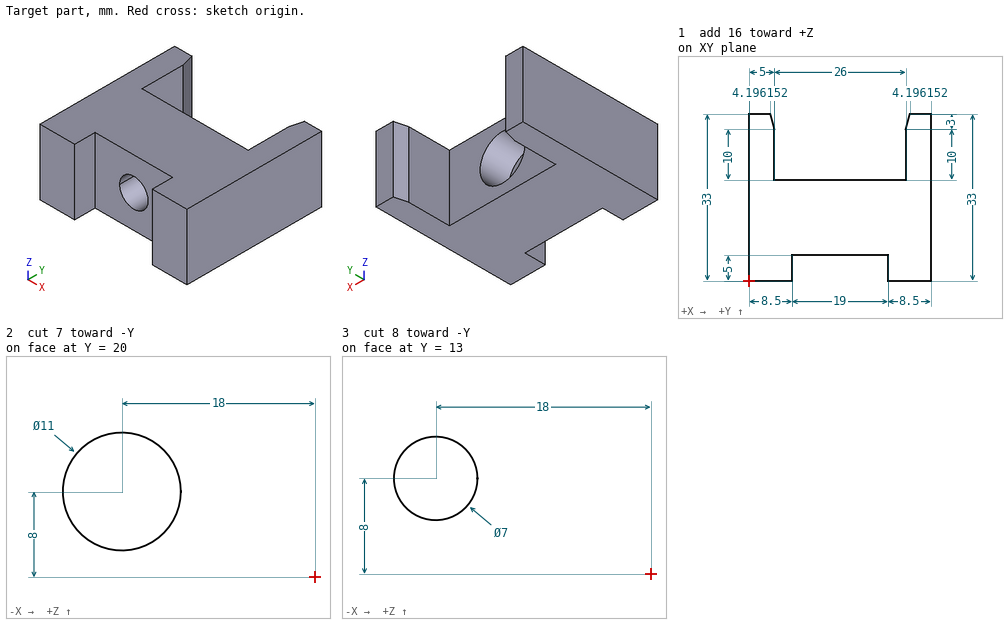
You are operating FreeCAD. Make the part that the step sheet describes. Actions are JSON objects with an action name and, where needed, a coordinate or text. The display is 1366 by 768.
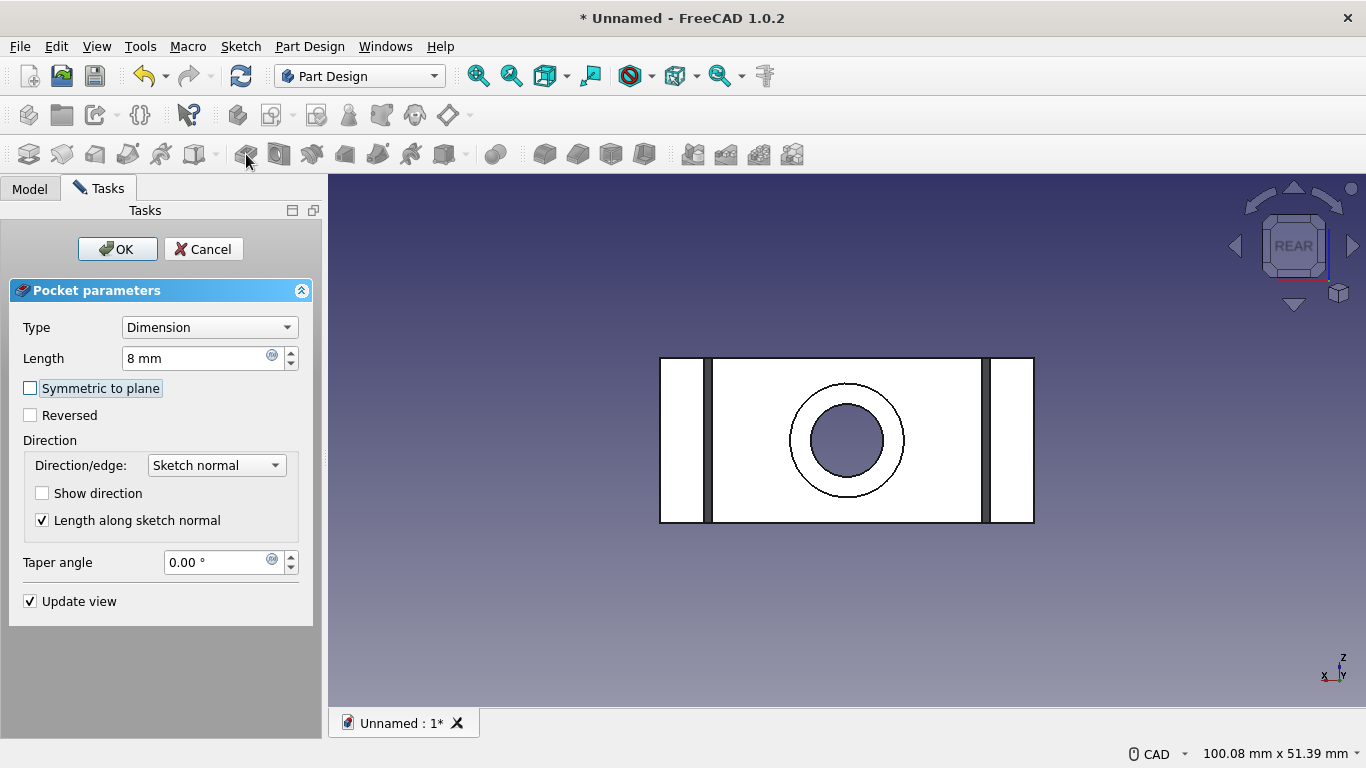
{"action": "left_click", "coordinate": [118, 249]}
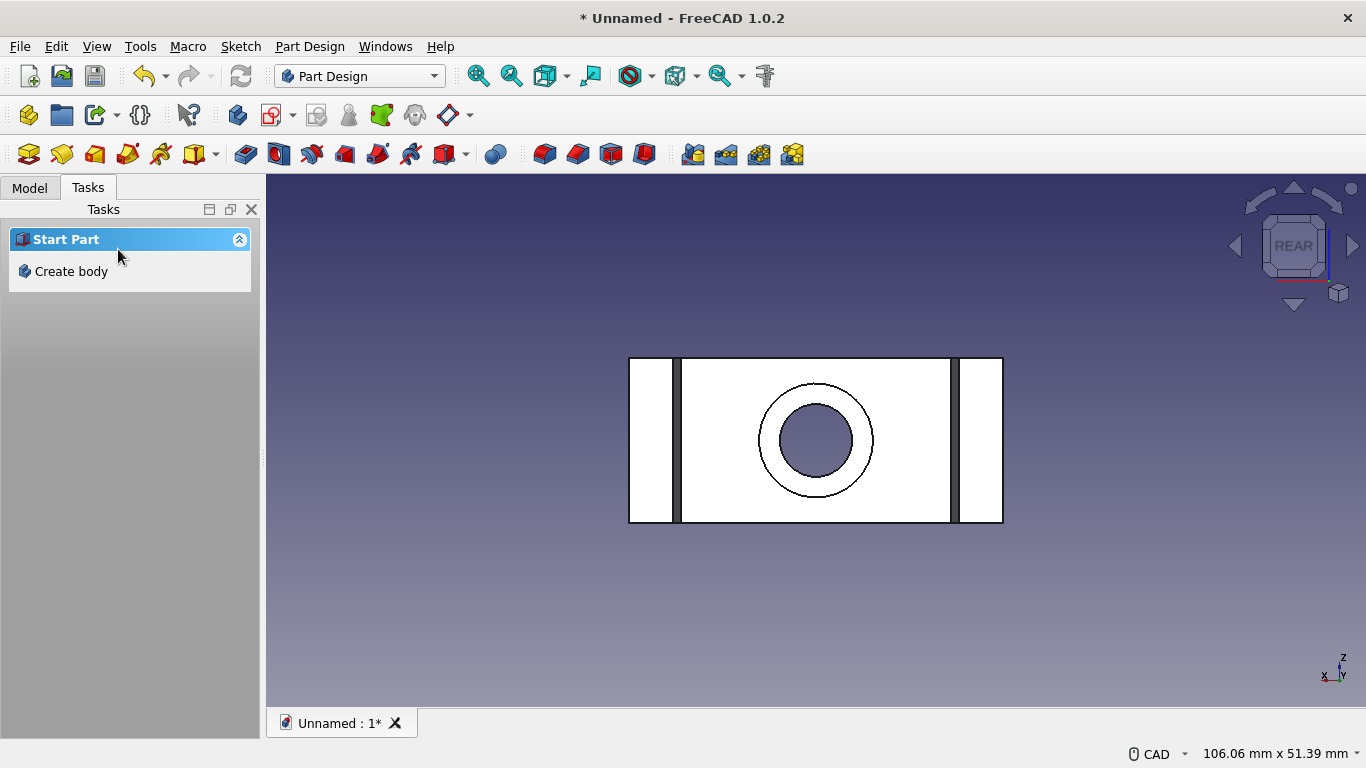
{"action": "key", "text": "0"}